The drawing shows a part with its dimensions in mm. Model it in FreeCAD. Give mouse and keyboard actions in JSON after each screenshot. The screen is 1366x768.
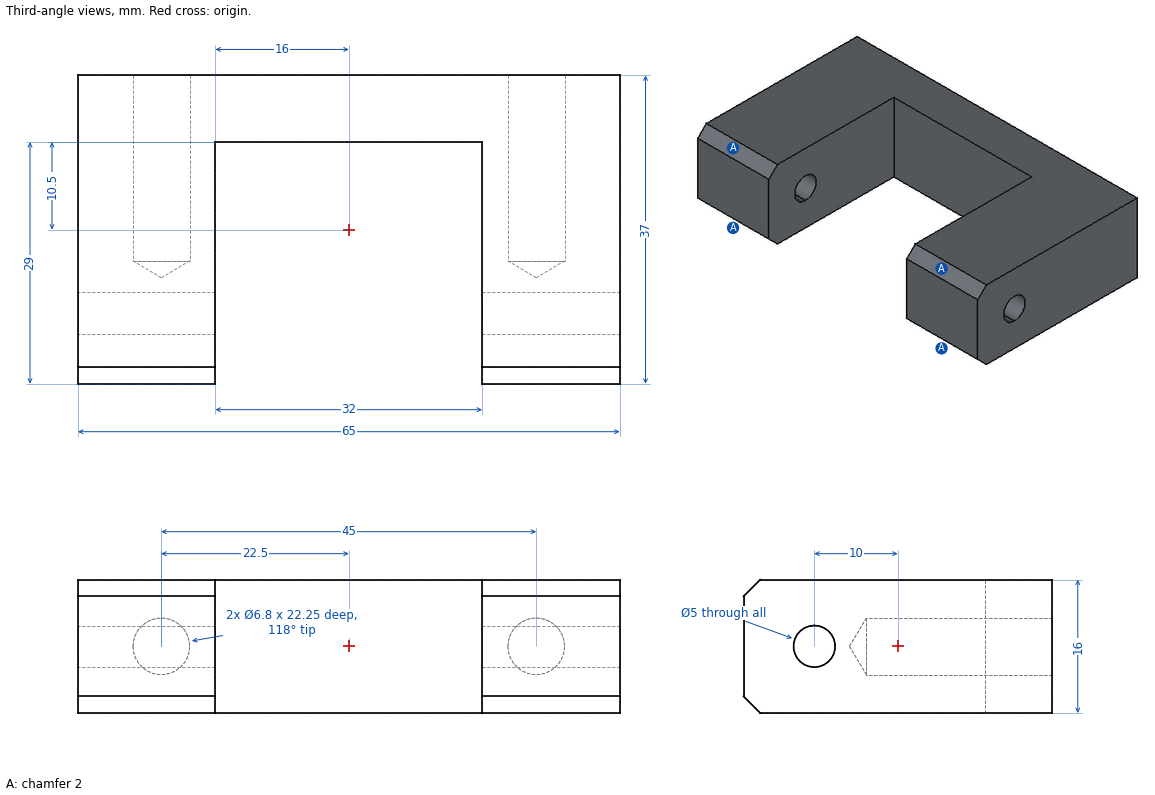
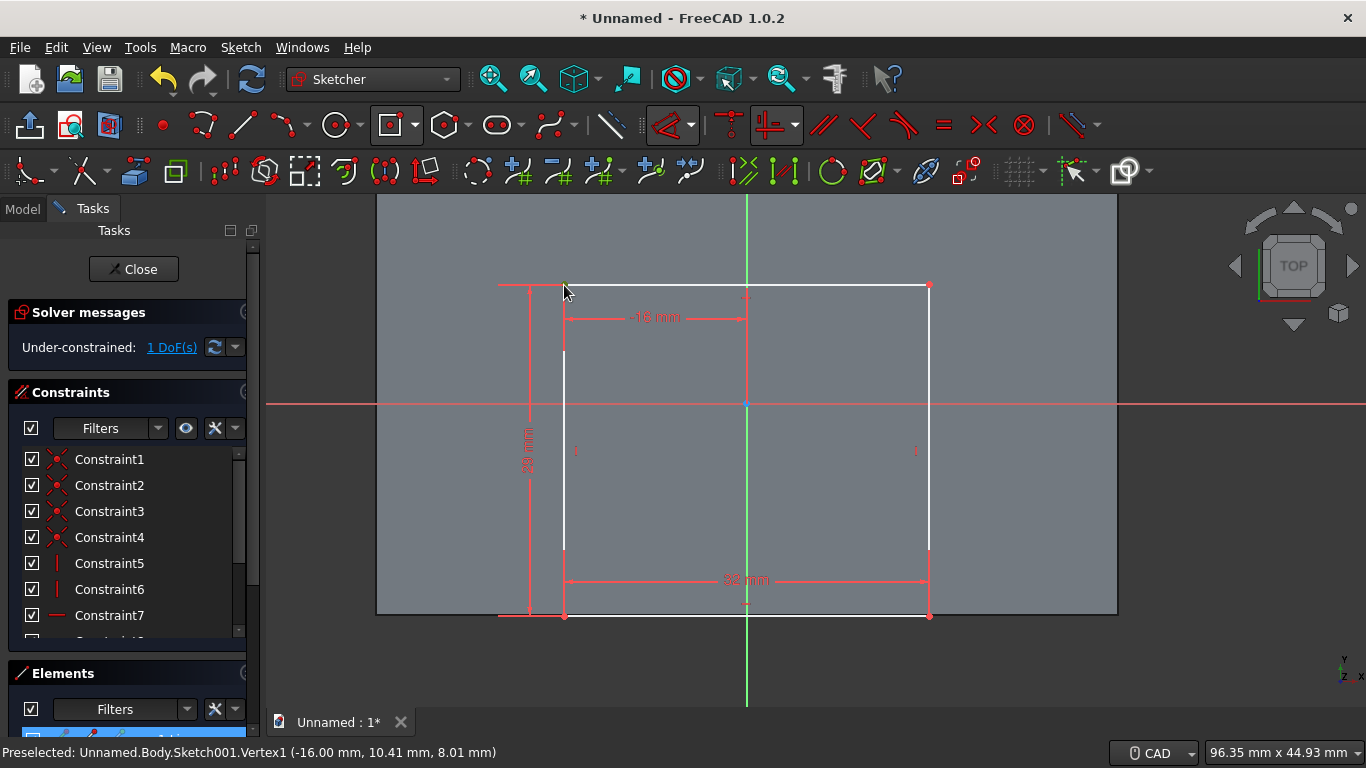
{"action": "key", "text": "i"}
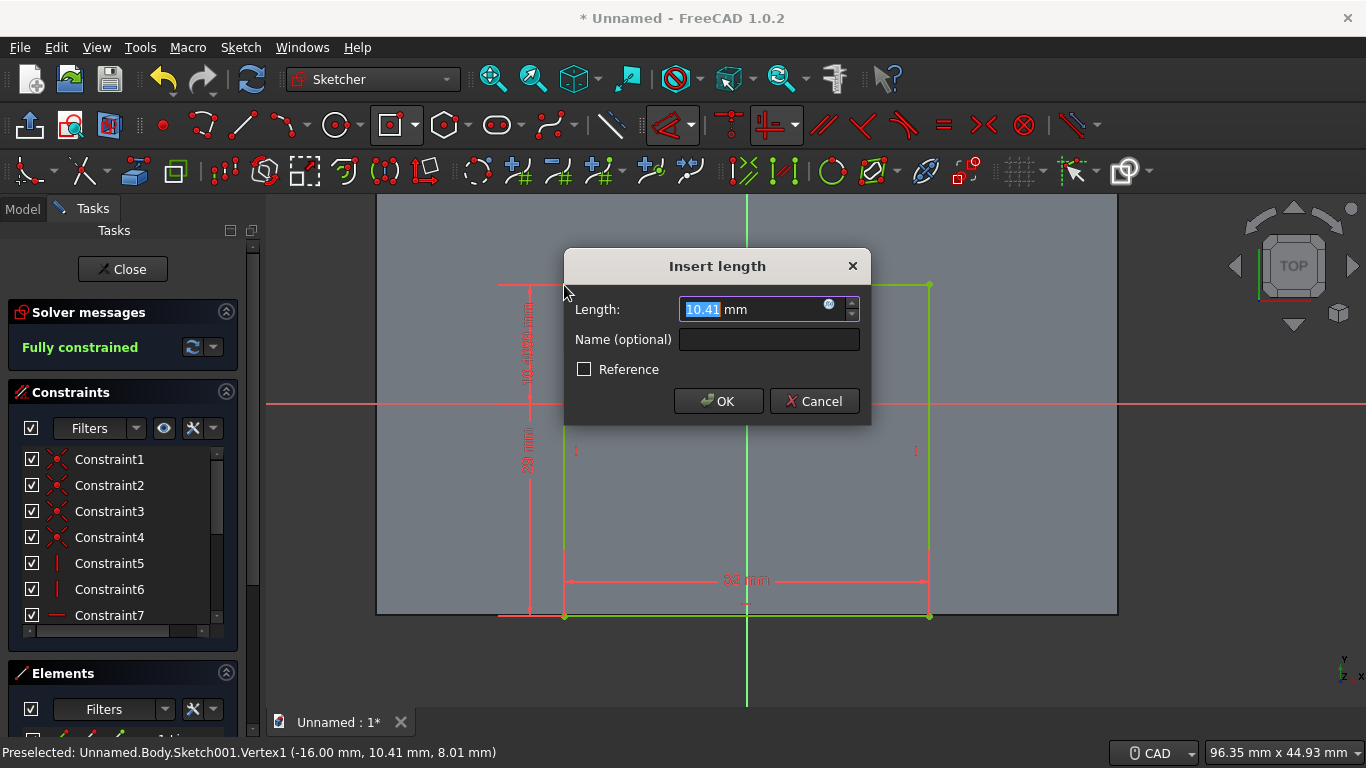
{"action": "type", "text": "10.5"}
{"action": "key", "text": "Return"}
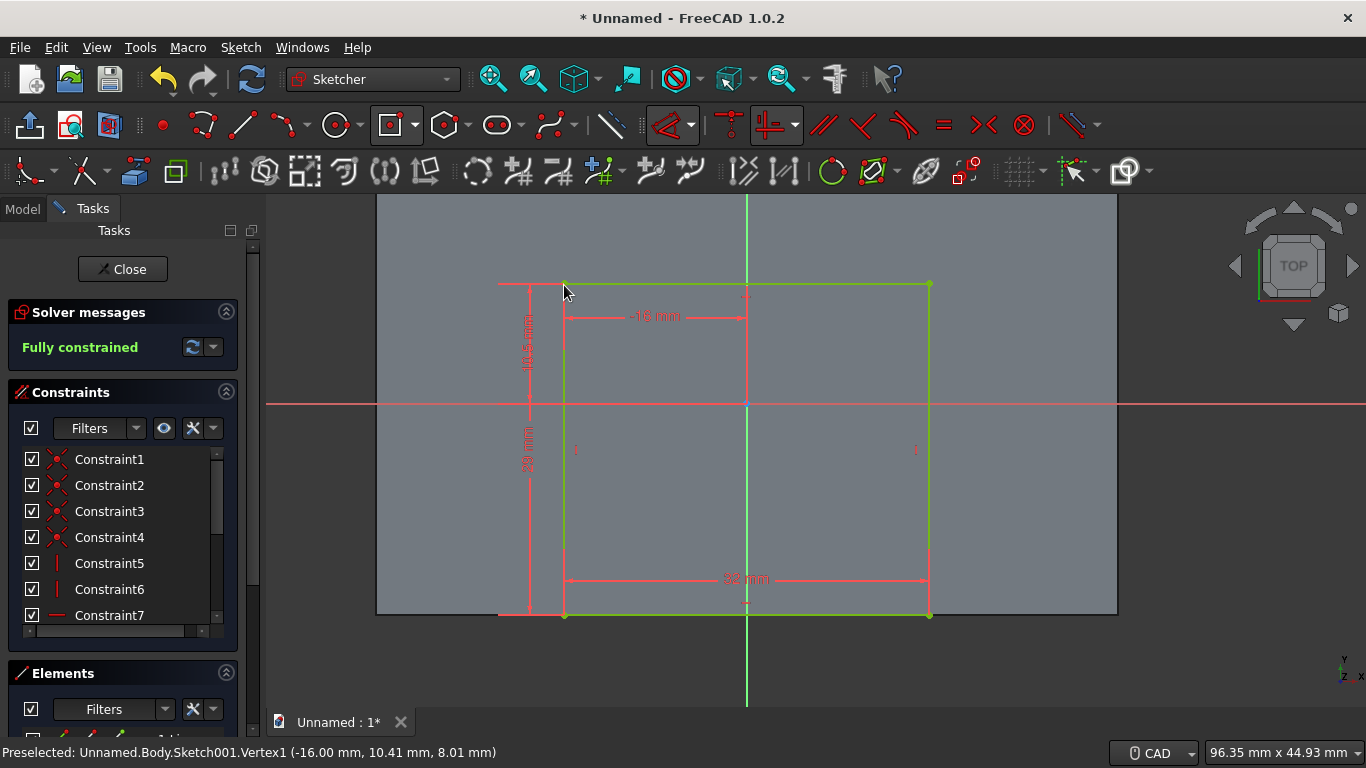
{"action": "left_click", "coordinate": [123, 269]}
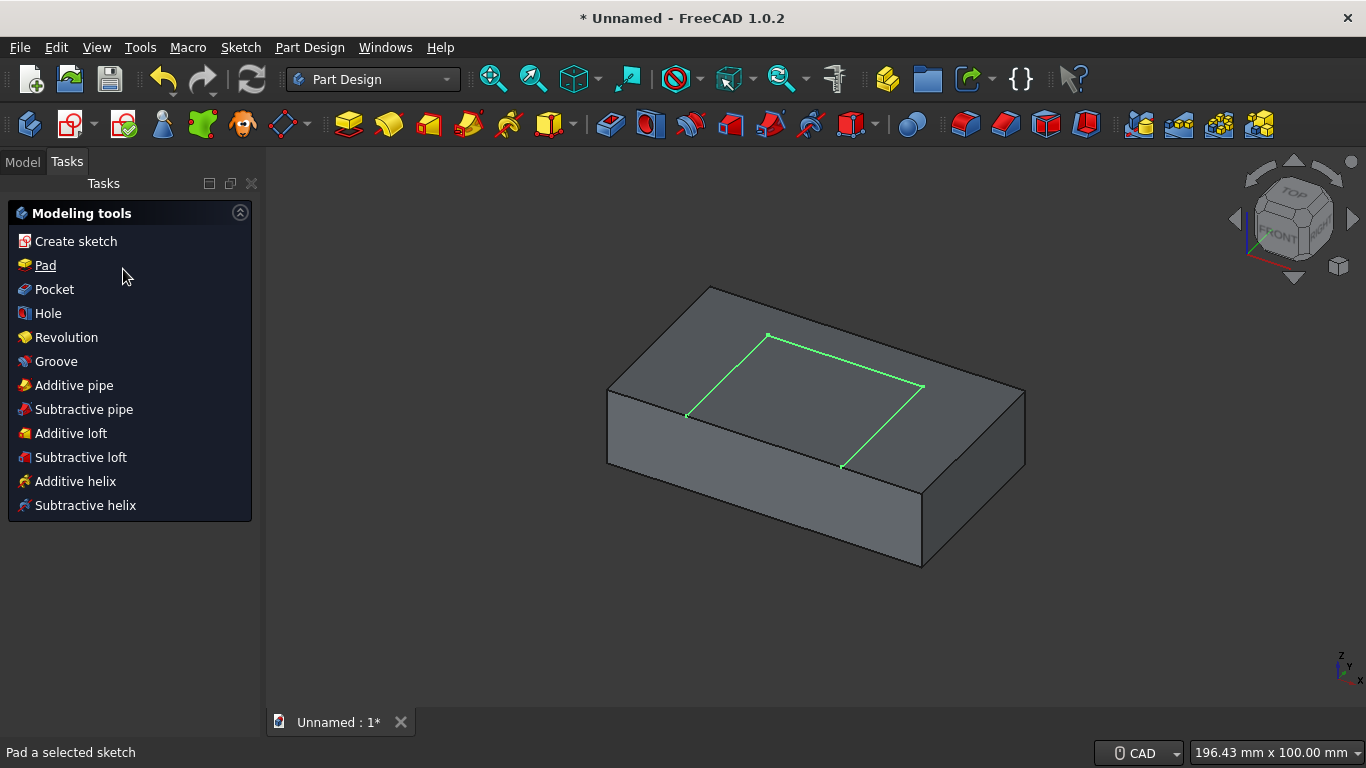
{"action": "left_click", "coordinate": [612, 124]}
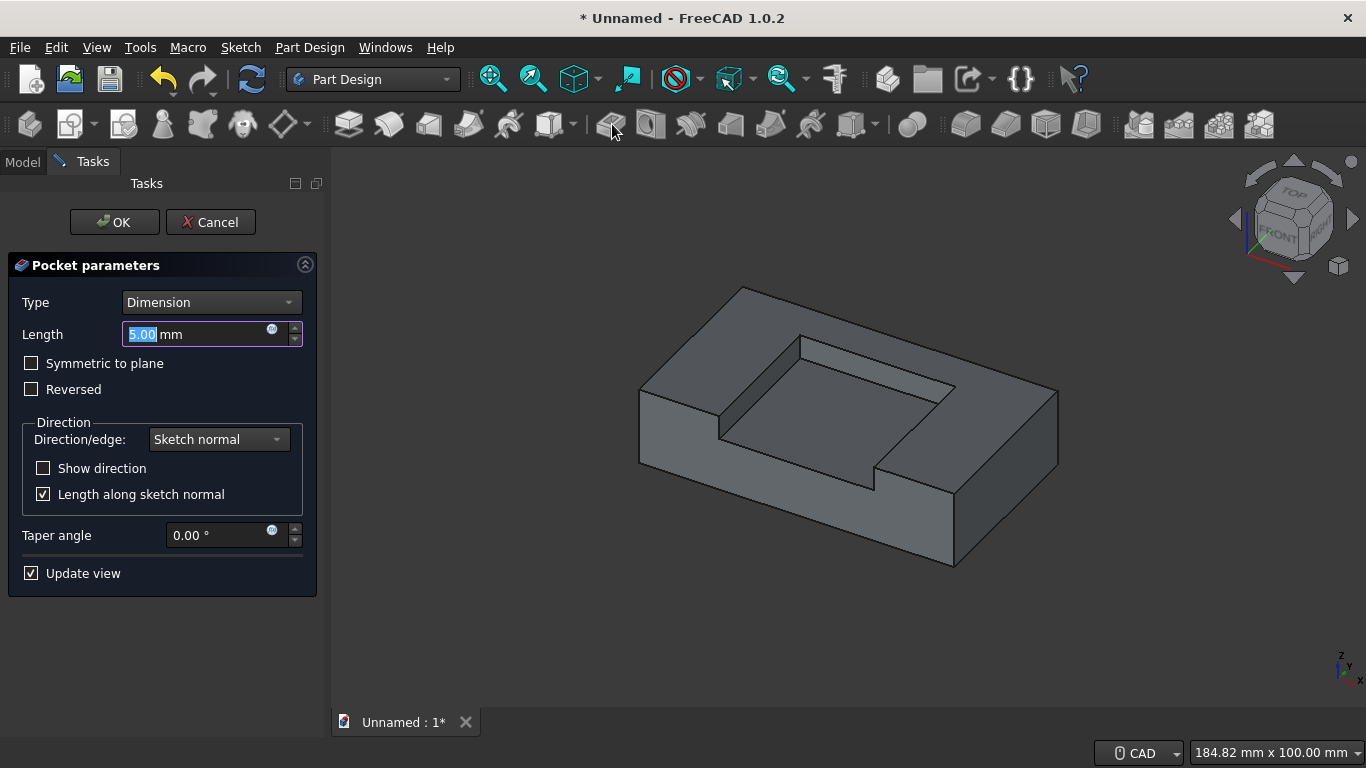
{"action": "left_click", "coordinate": [212, 302]}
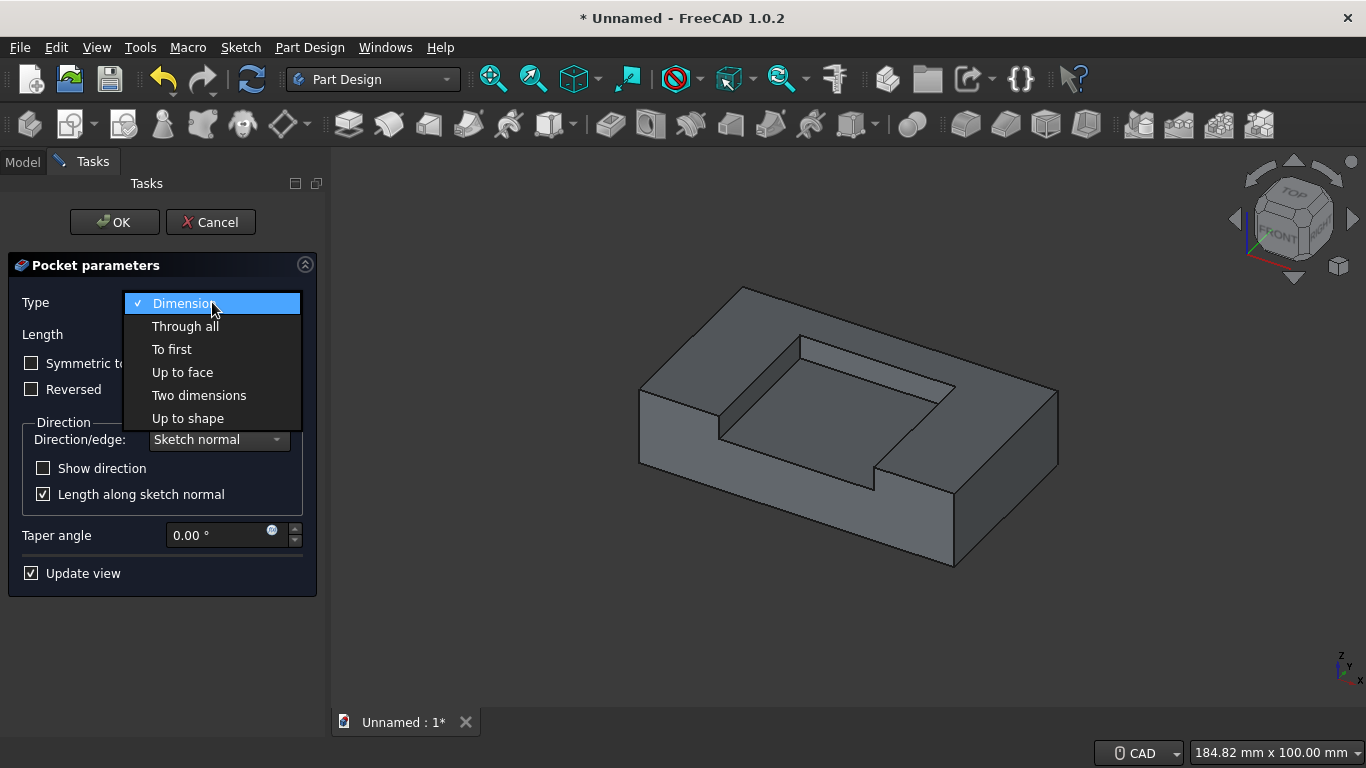
{"action": "left_click", "coordinate": [212, 326]}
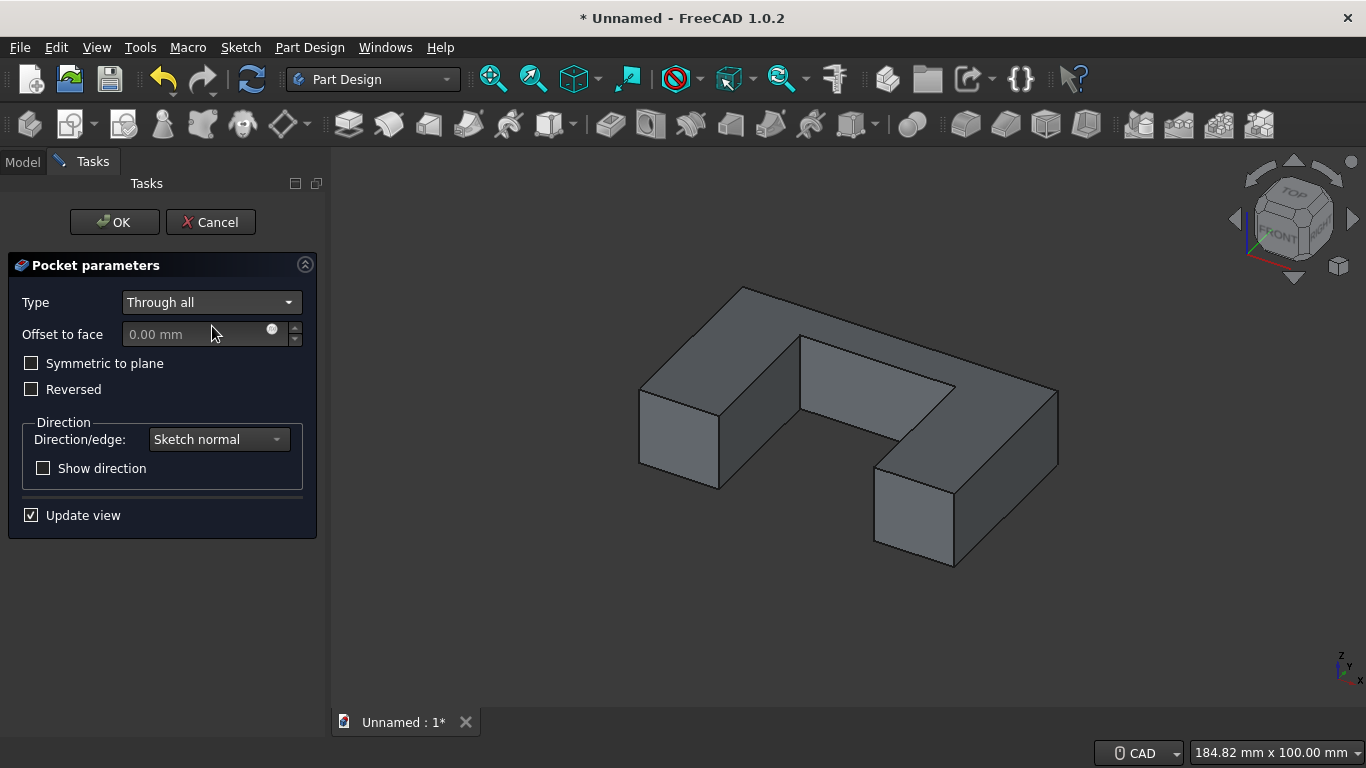
{"action": "left_click", "coordinate": [115, 222]}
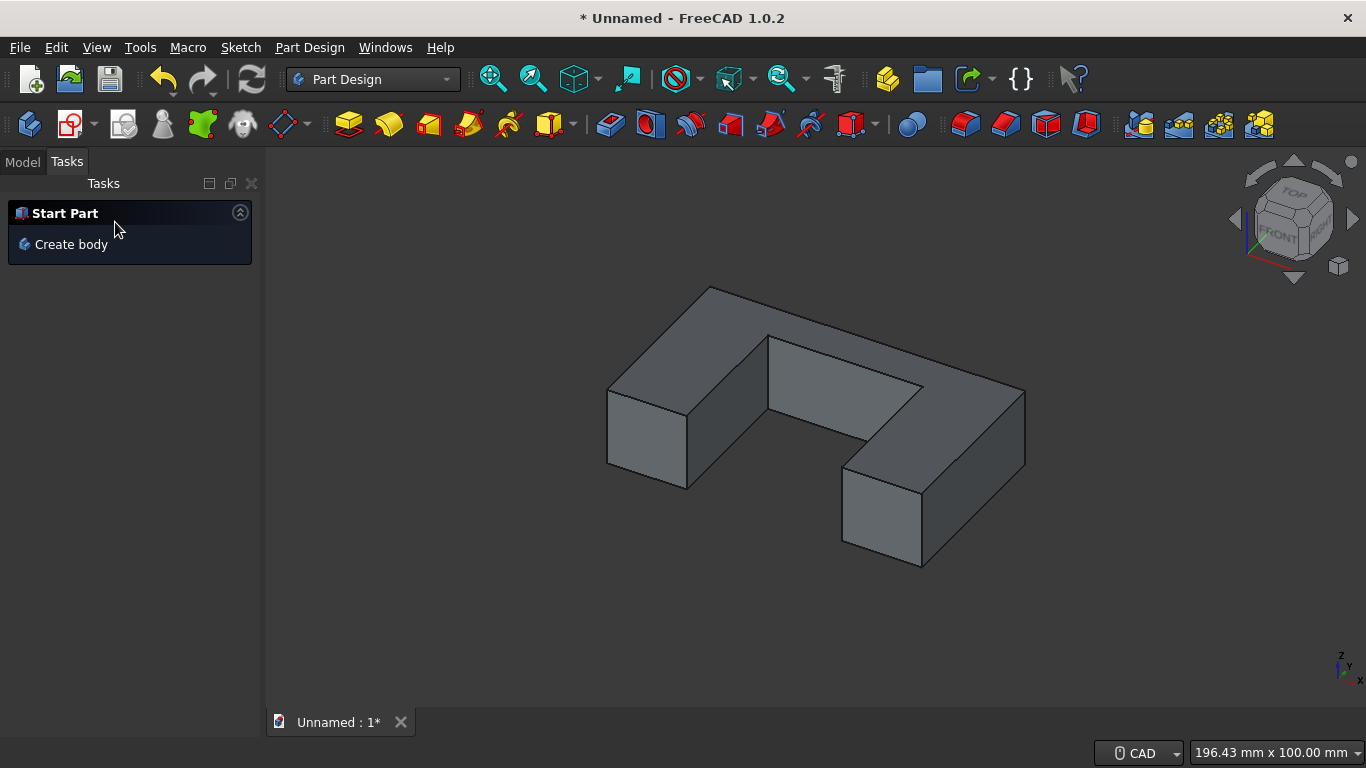
{"action": "left_click", "coordinate": [988, 463]}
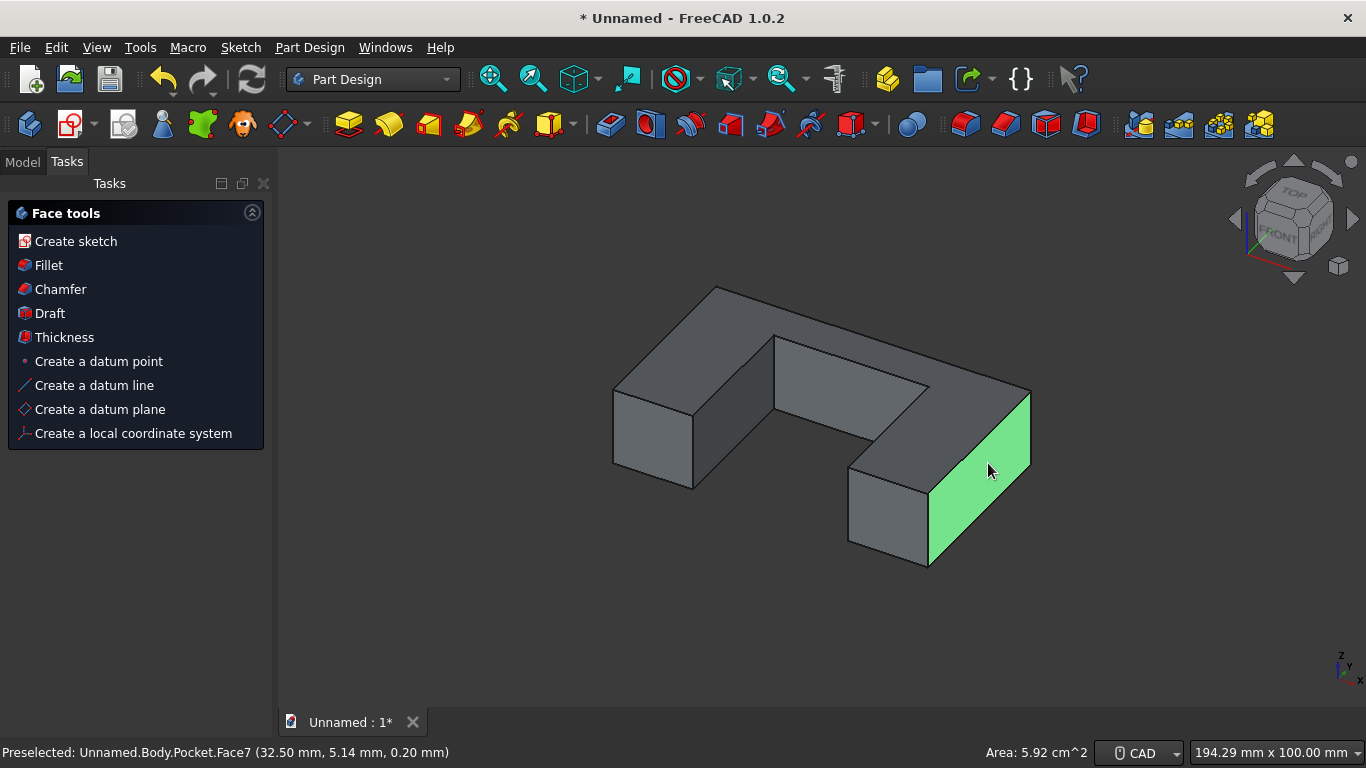
{"action": "left_click", "coordinate": [70, 124]}